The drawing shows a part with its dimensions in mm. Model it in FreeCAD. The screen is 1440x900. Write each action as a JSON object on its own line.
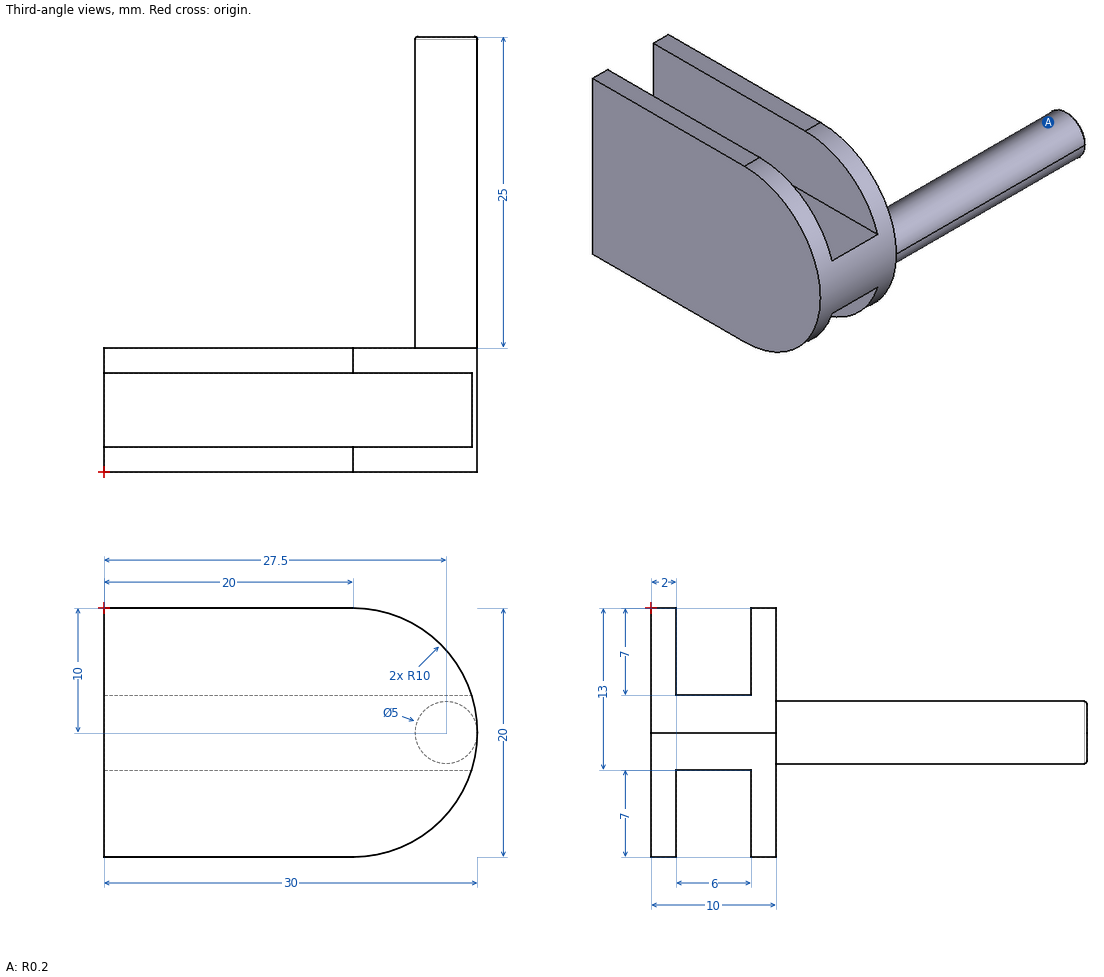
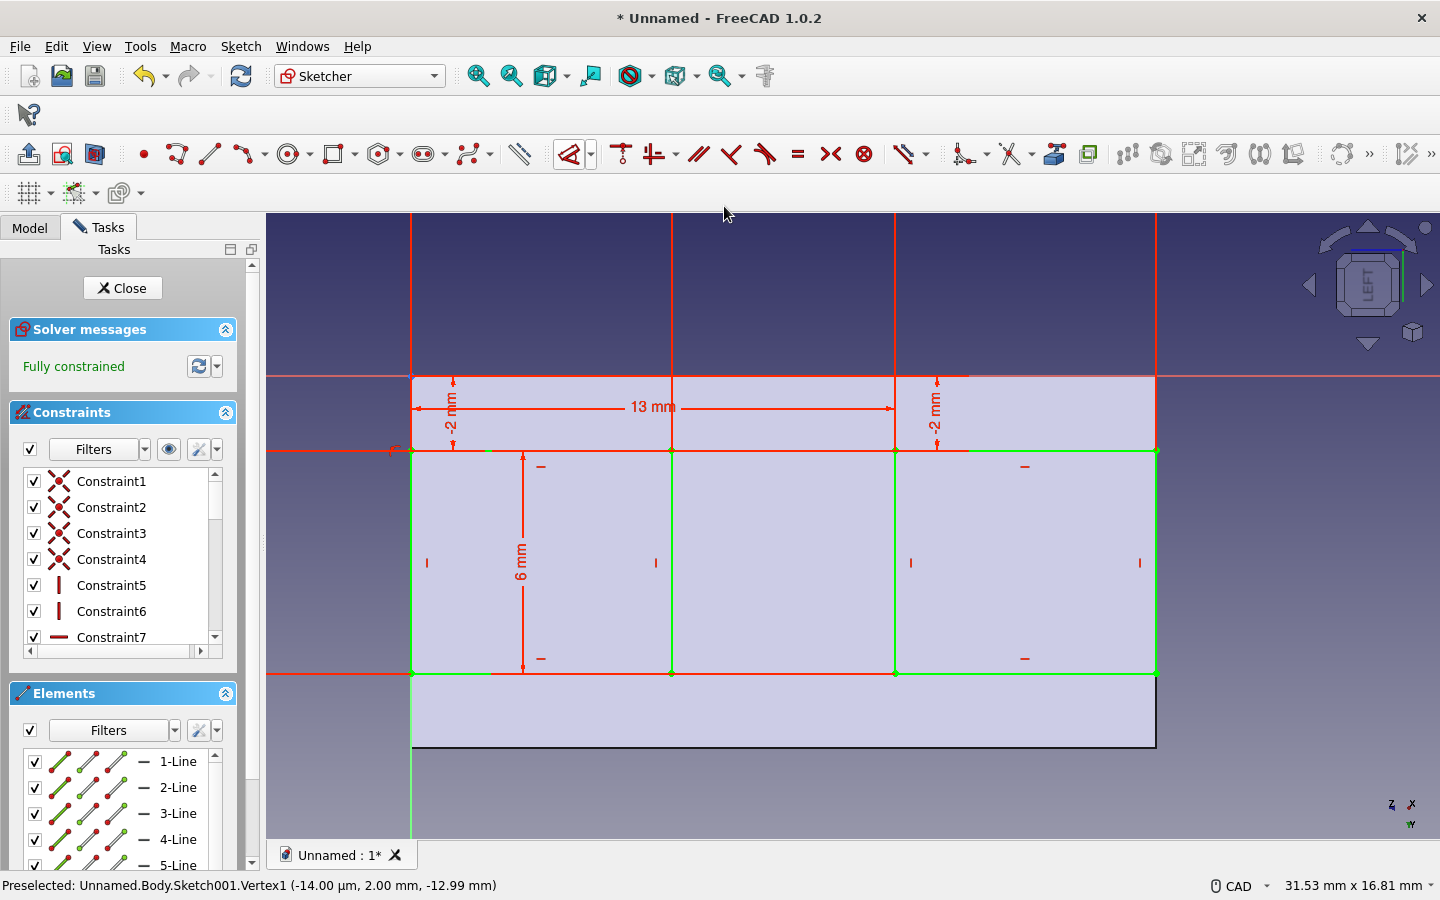
{"action": "left_click", "coordinate": [123, 288]}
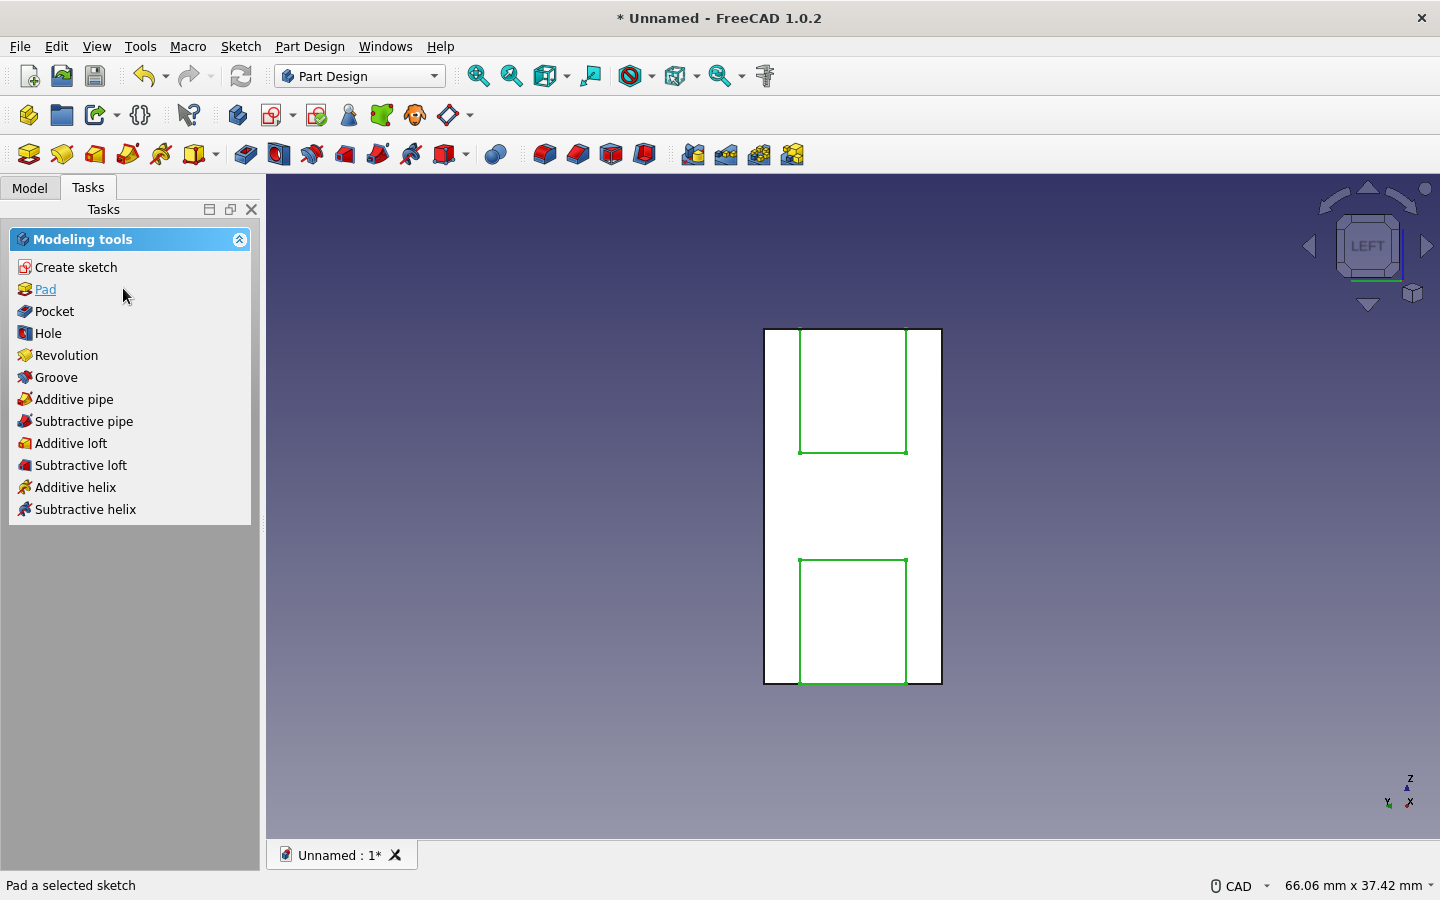
{"action": "left_click", "coordinate": [246, 154]}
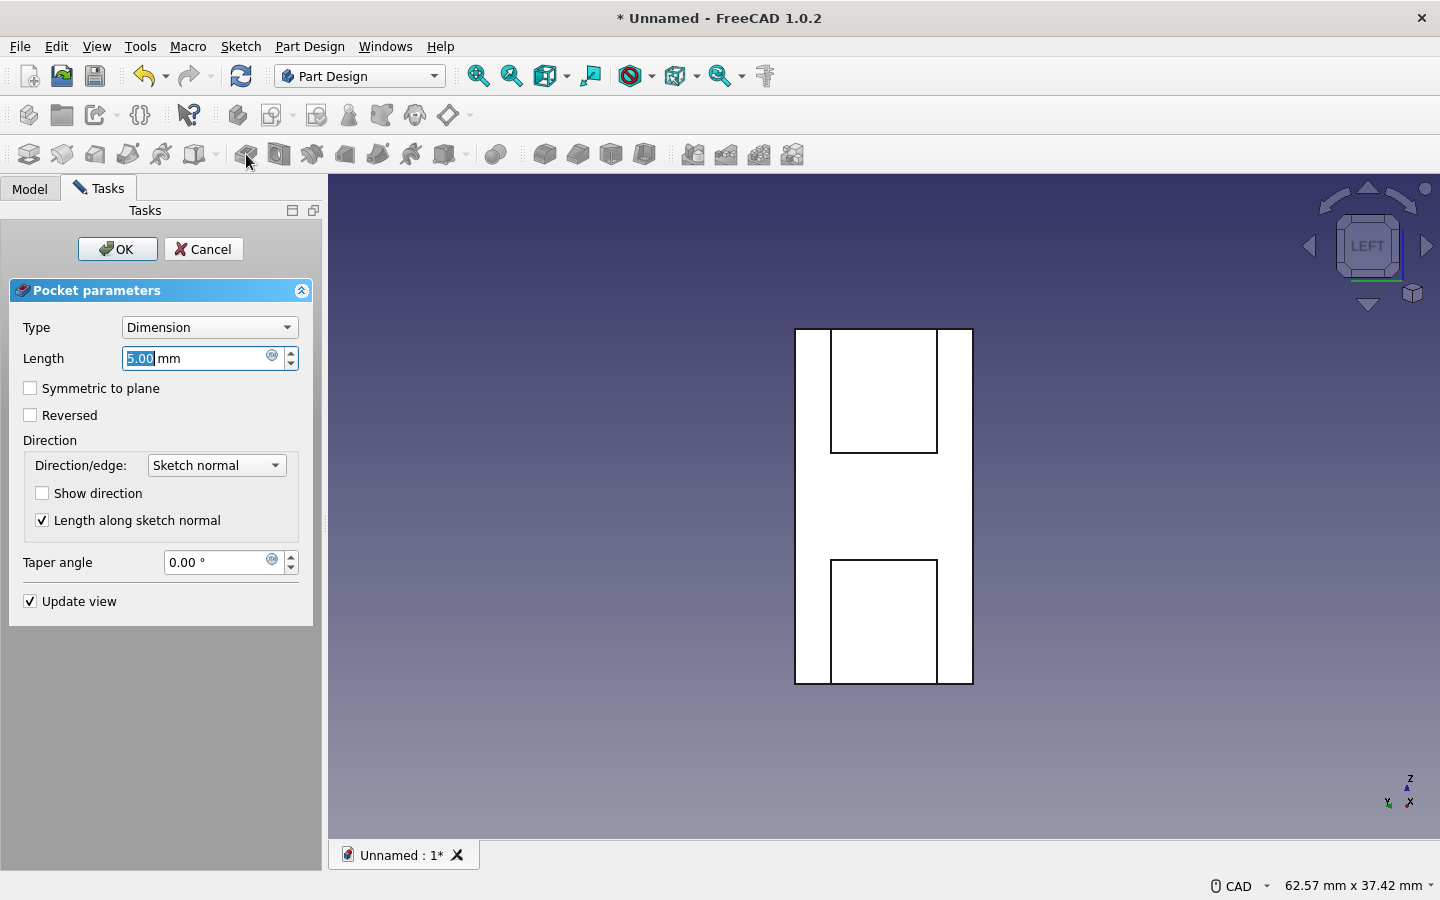
{"action": "left_click", "coordinate": [210, 328]}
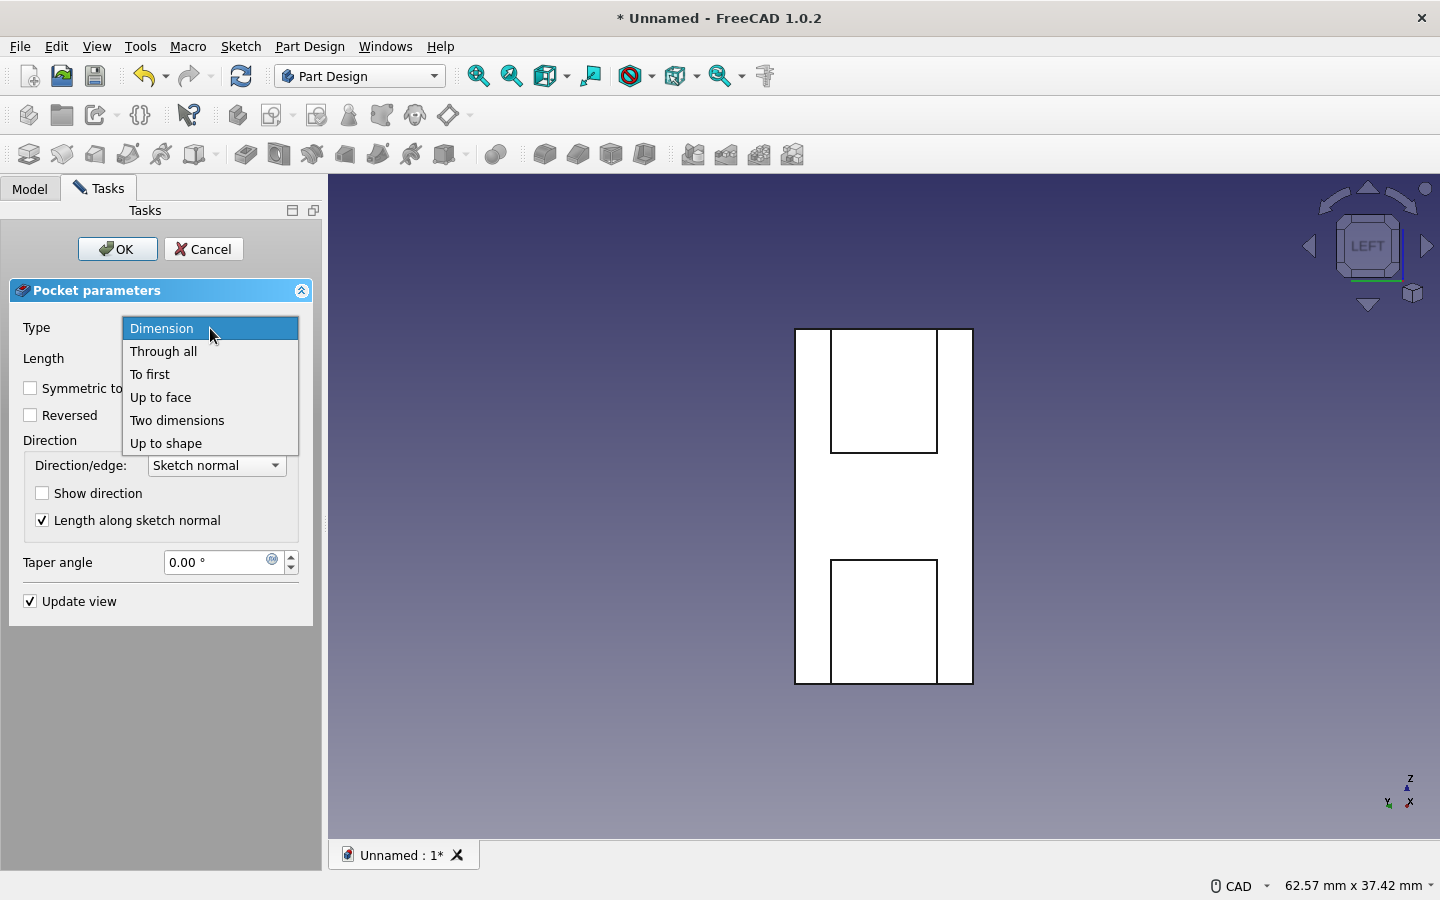
{"action": "left_click", "coordinate": [208, 352]}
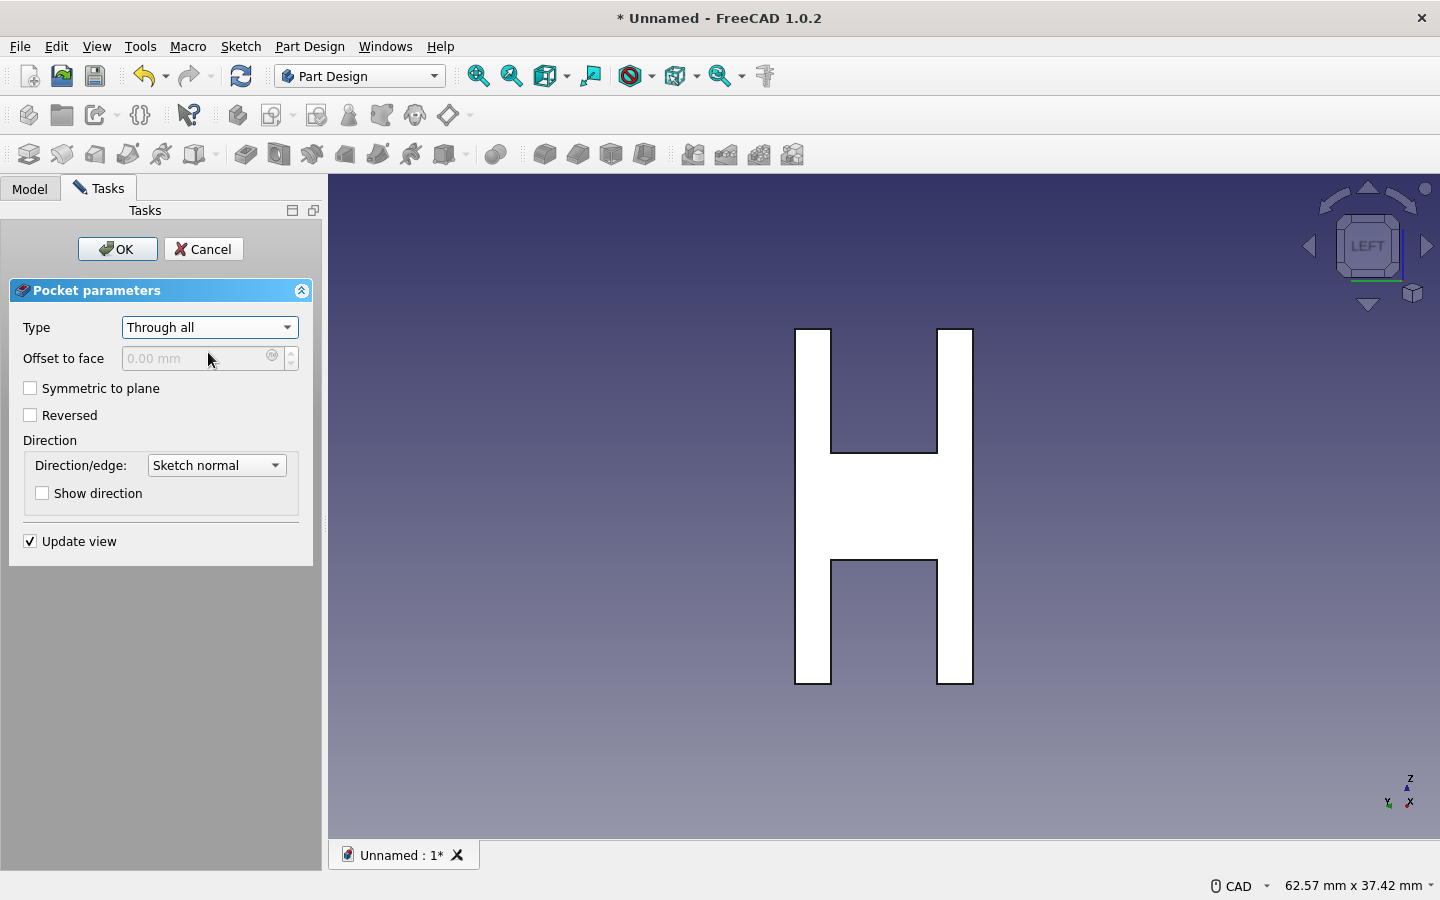
{"action": "left_click", "coordinate": [118, 249]}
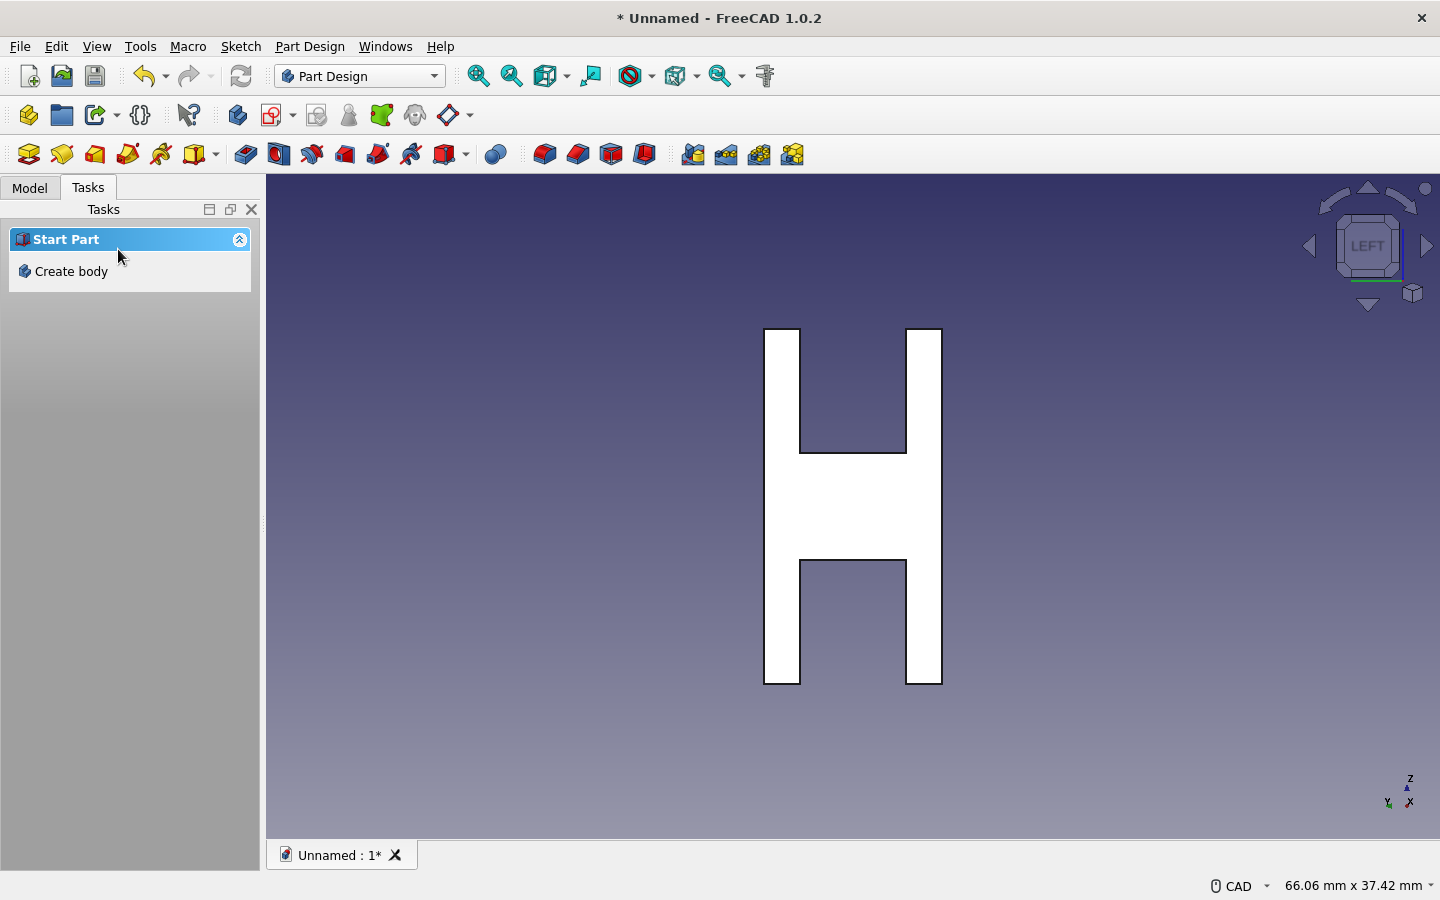
{"action": "key", "text": "4"}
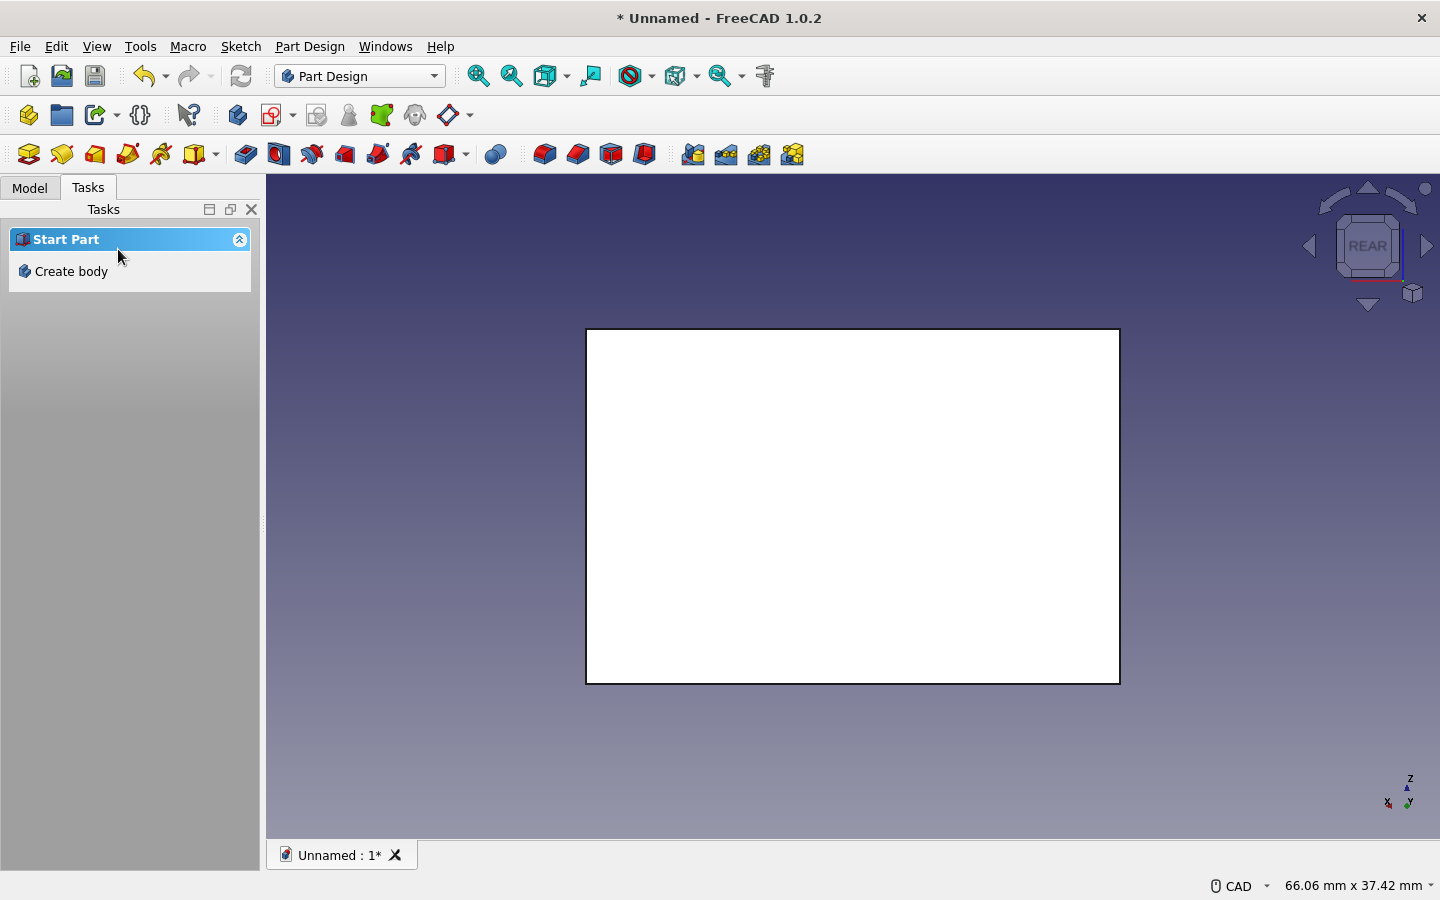
{"action": "left_click", "coordinate": [777, 506]}